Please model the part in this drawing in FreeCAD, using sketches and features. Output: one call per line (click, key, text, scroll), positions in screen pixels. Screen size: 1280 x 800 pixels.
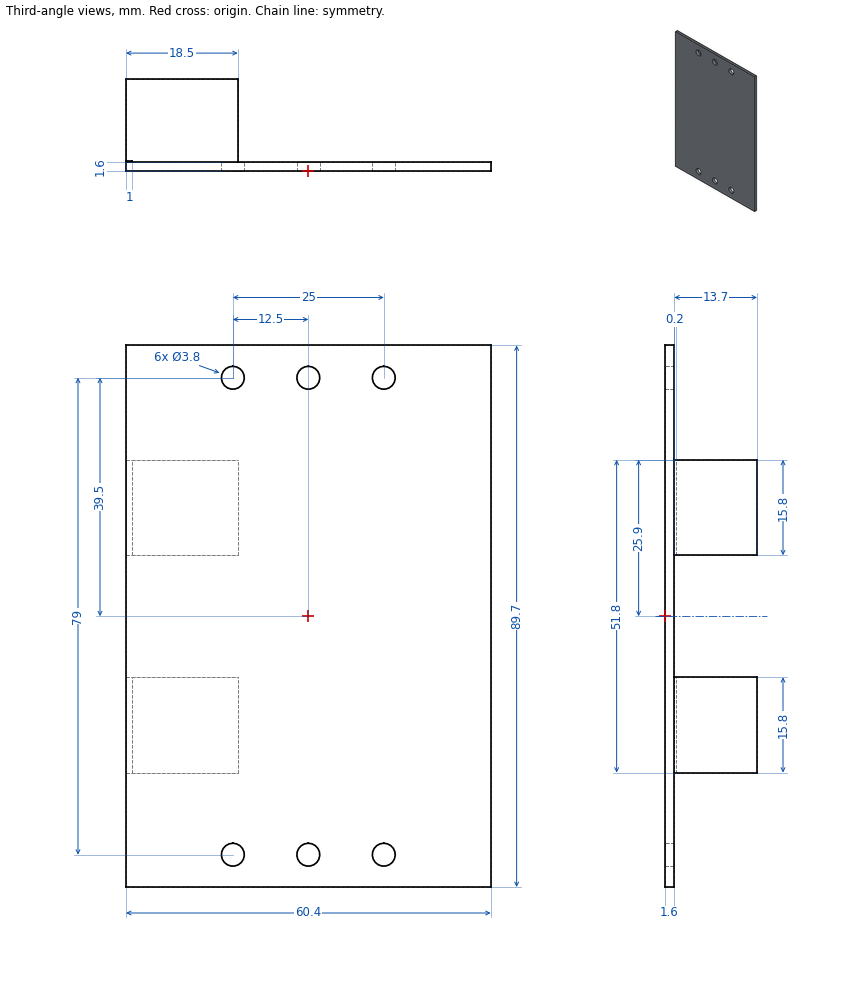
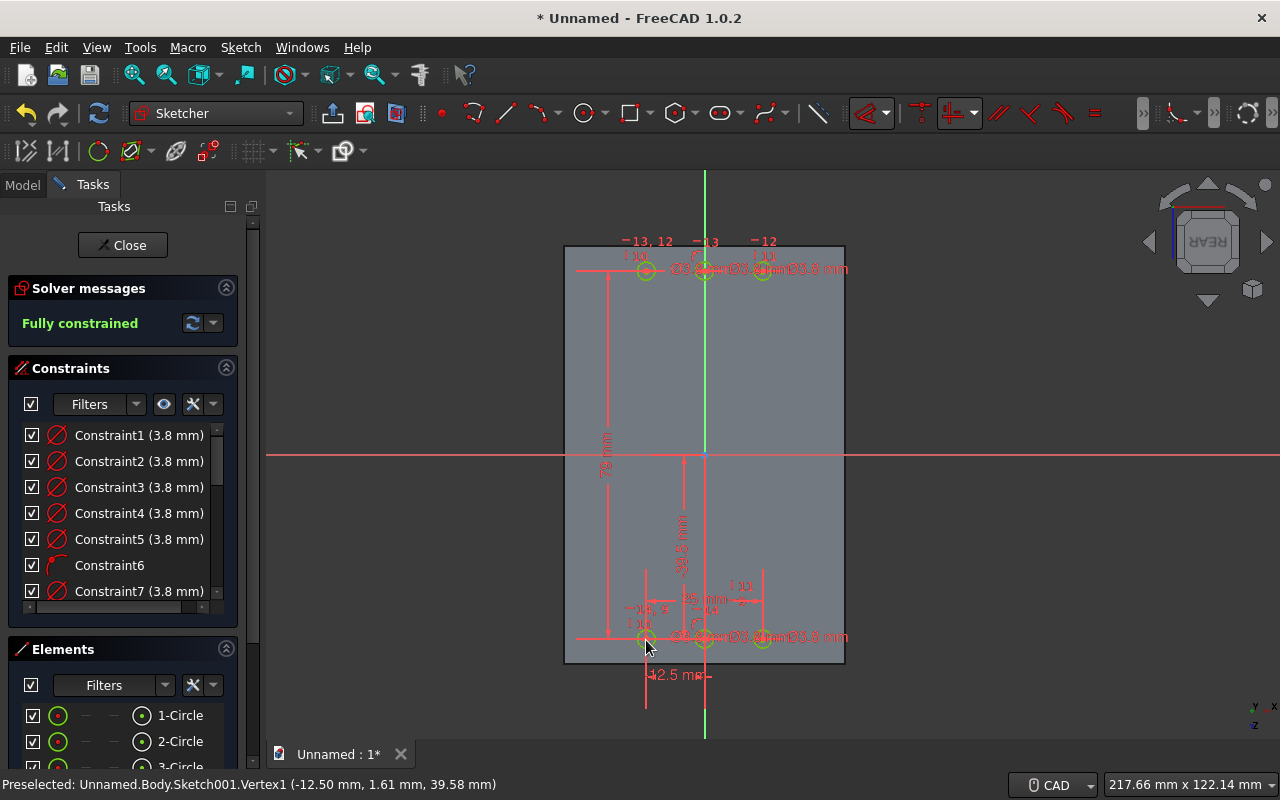
click(123, 245)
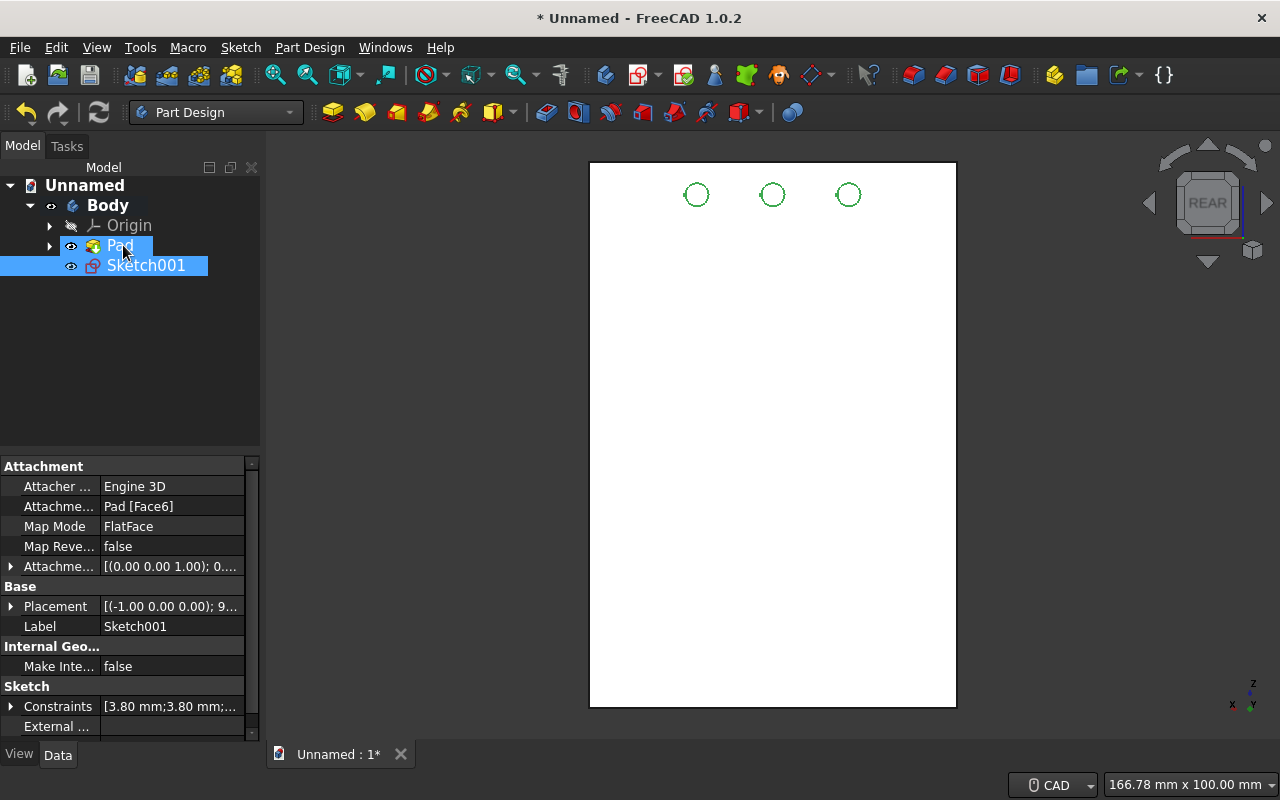
click(548, 112)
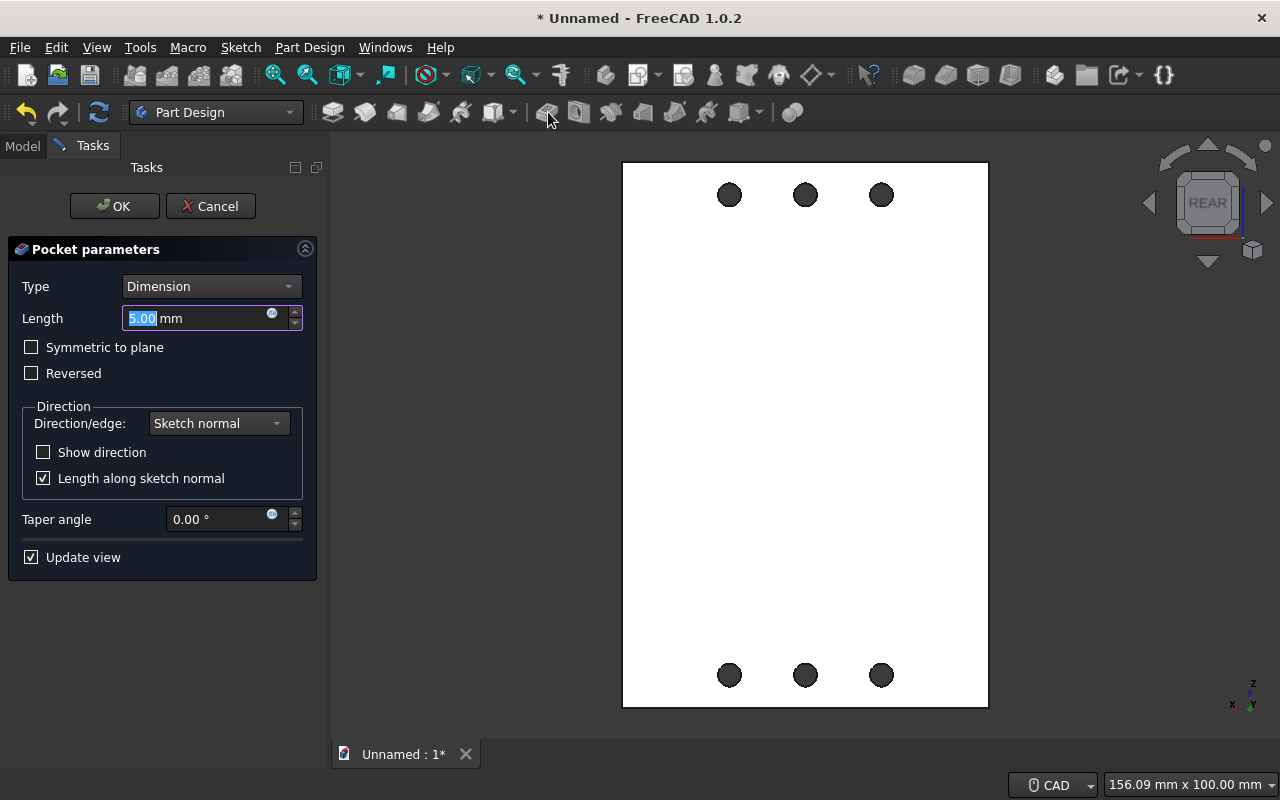
text(1.6)
key(Tab)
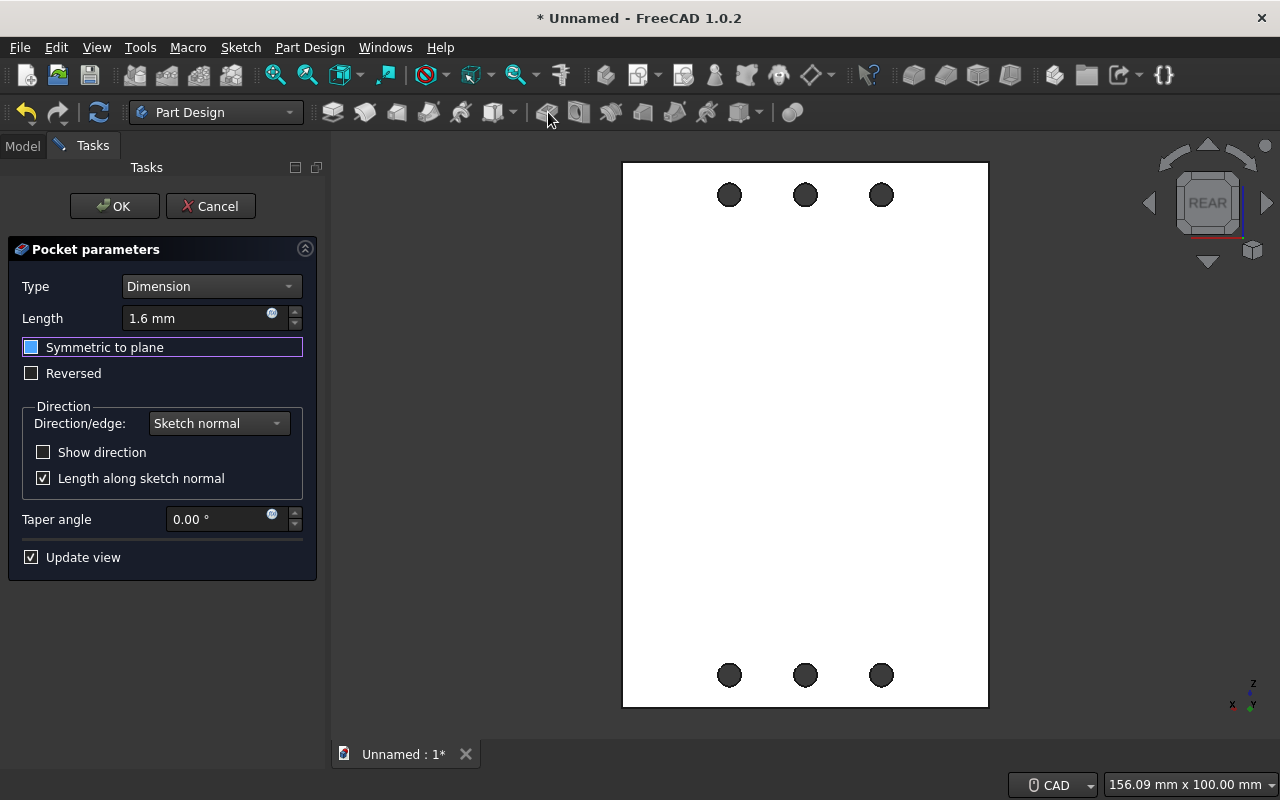
click(115, 206)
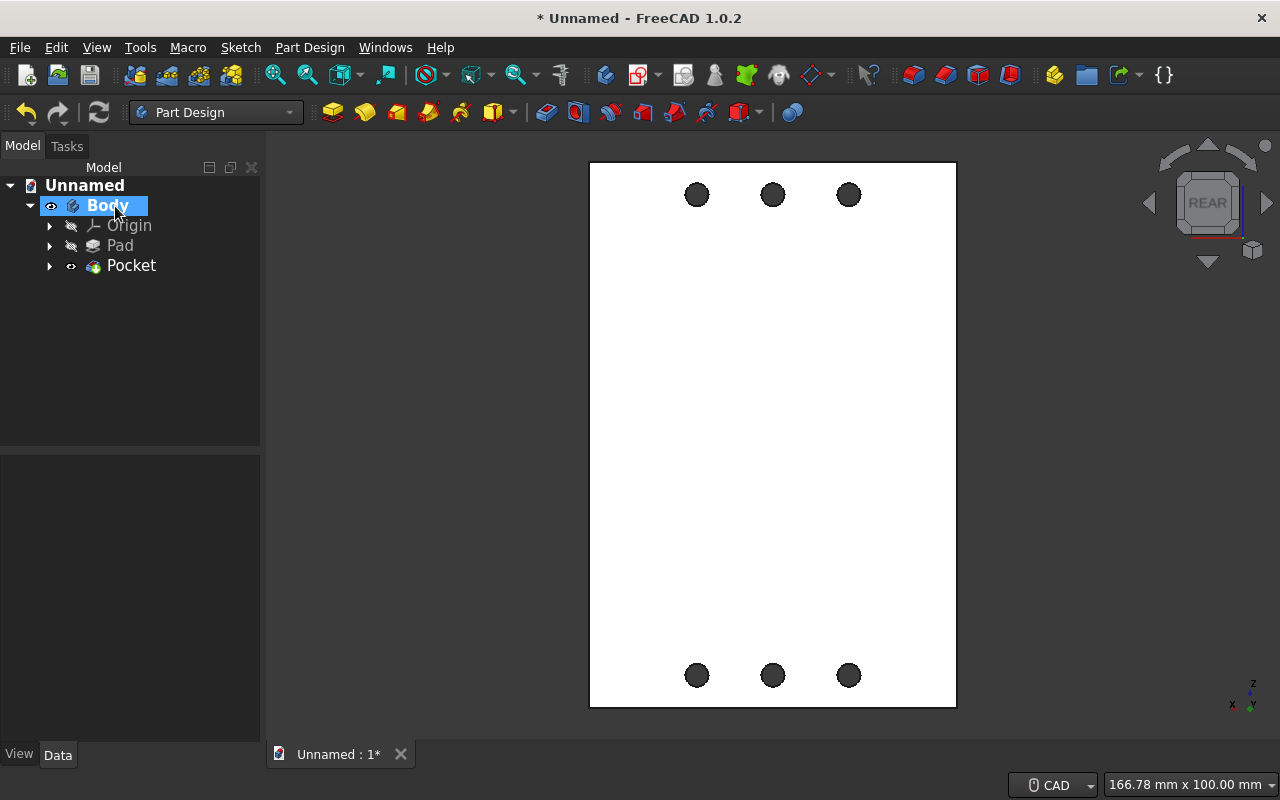
key(6)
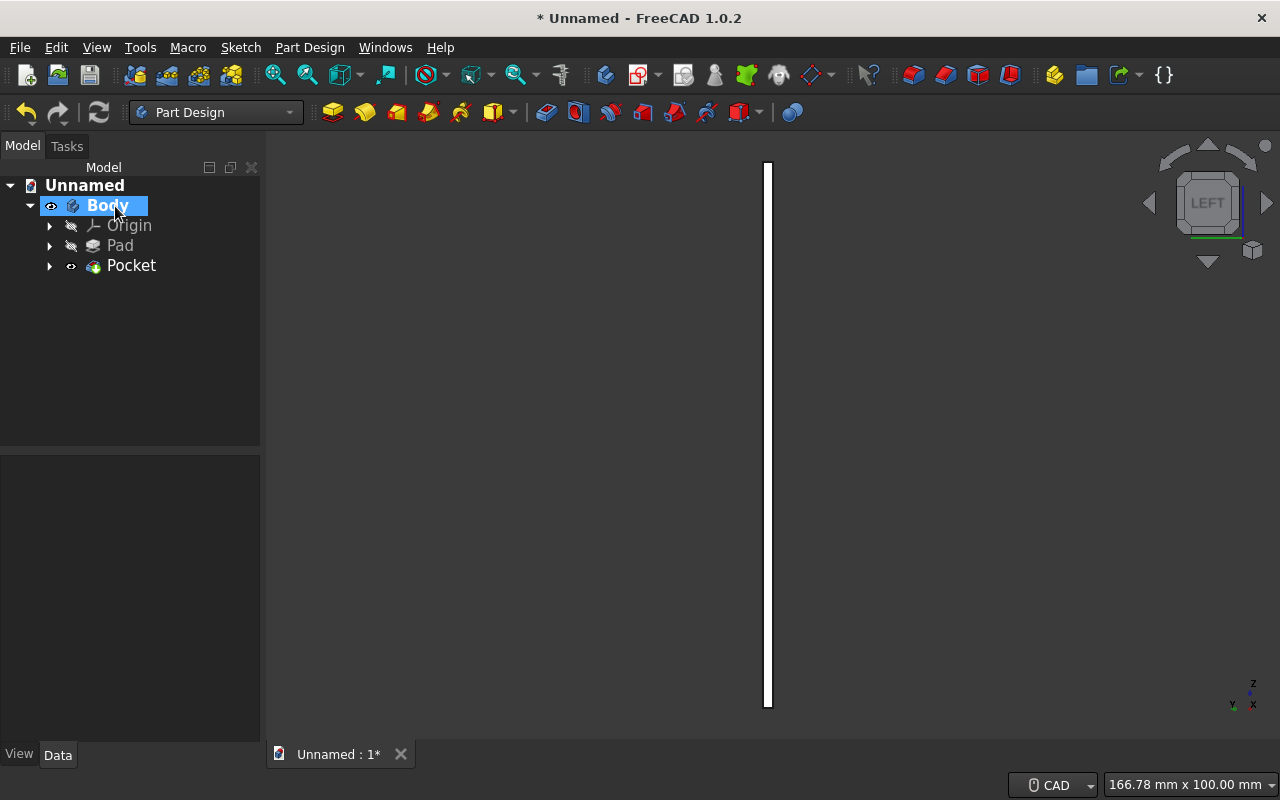
scroll(768, 278, up, 5)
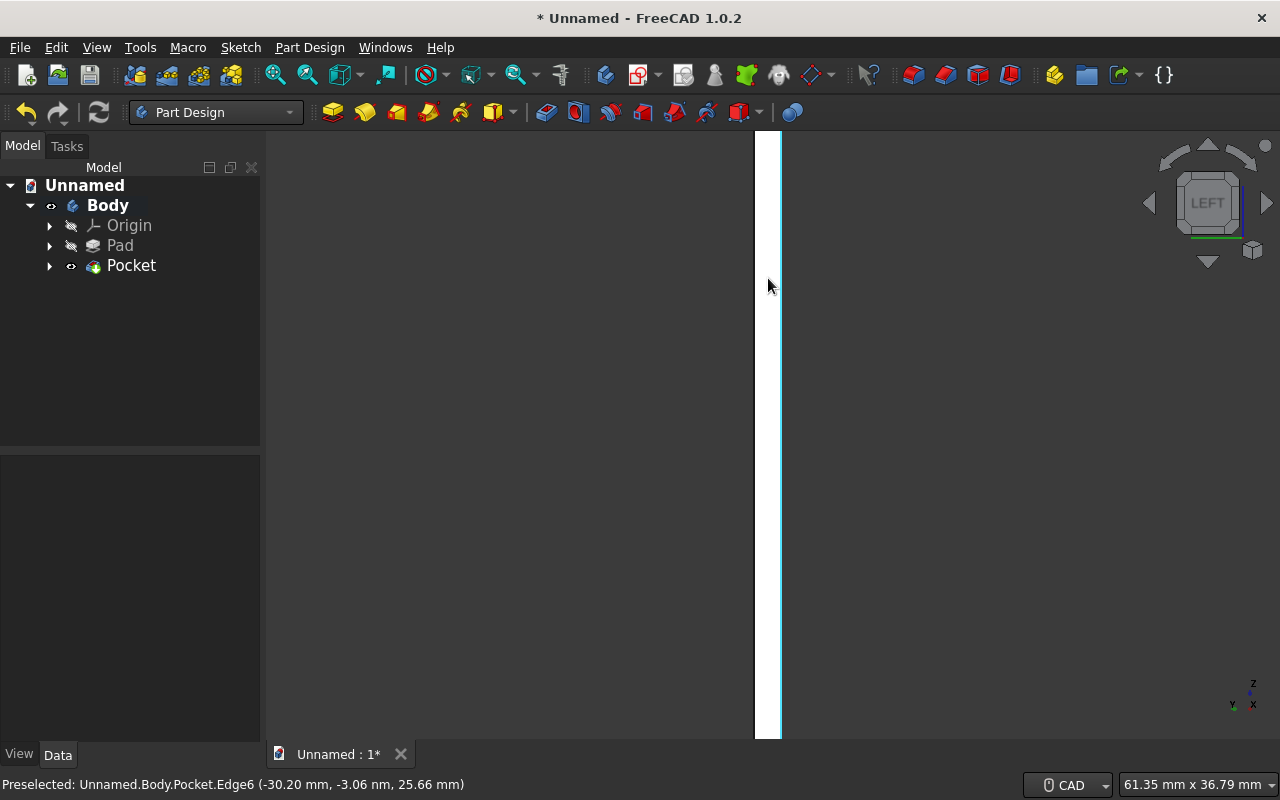
click(768, 280)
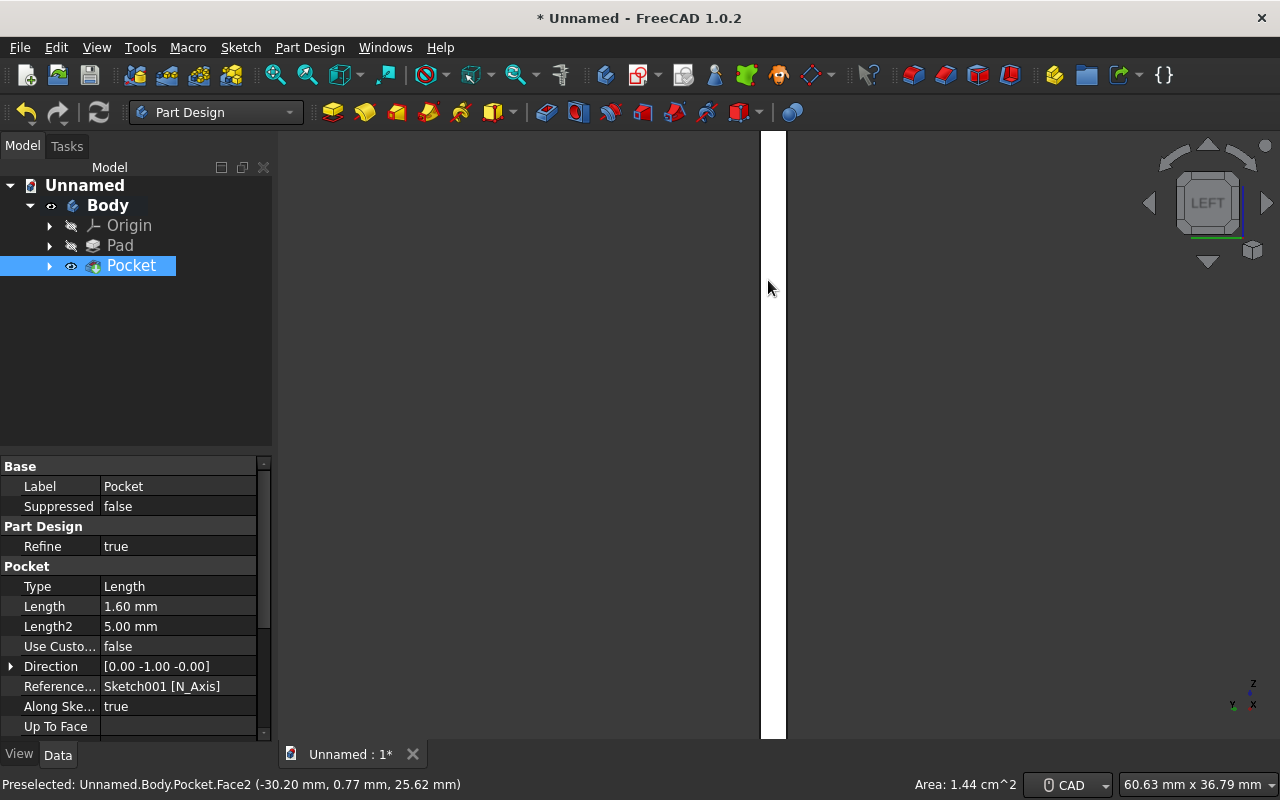
click(638, 76)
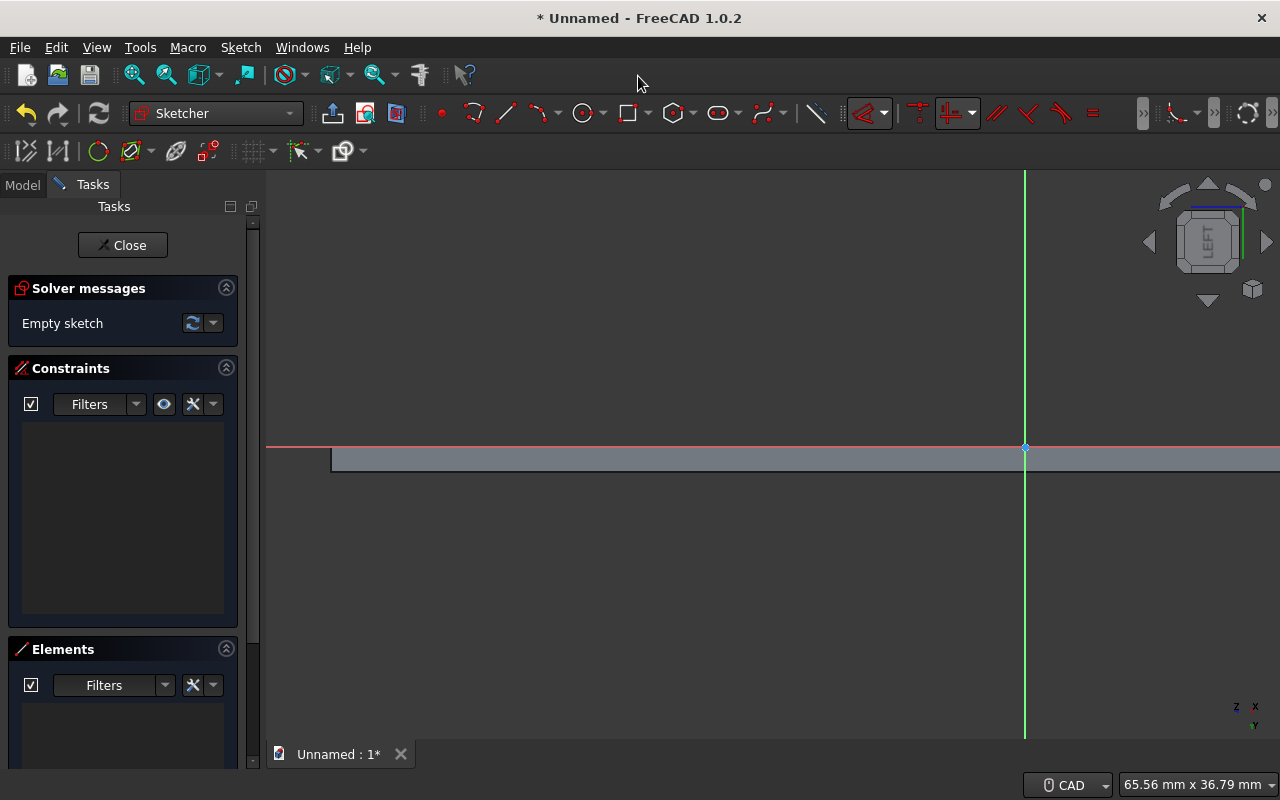
scroll(294, 229, down, 2)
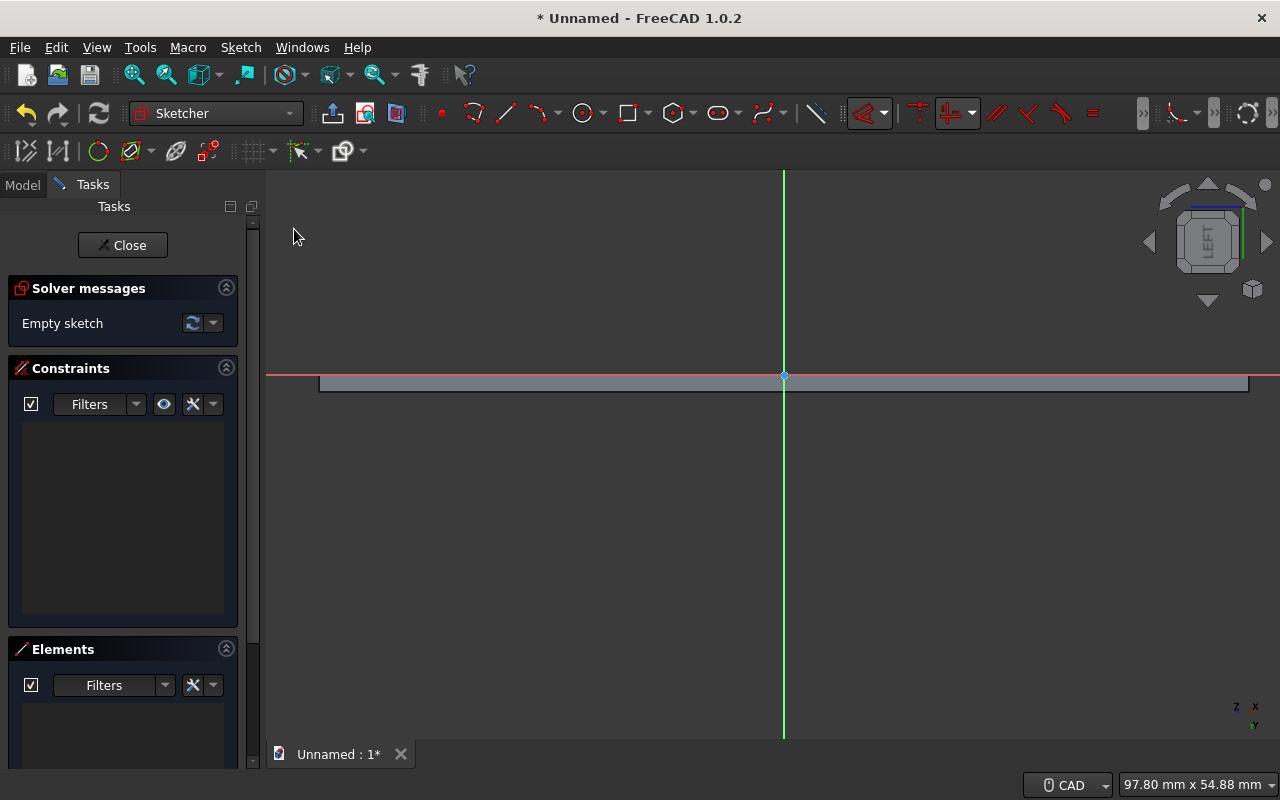
key(g)
key(r)